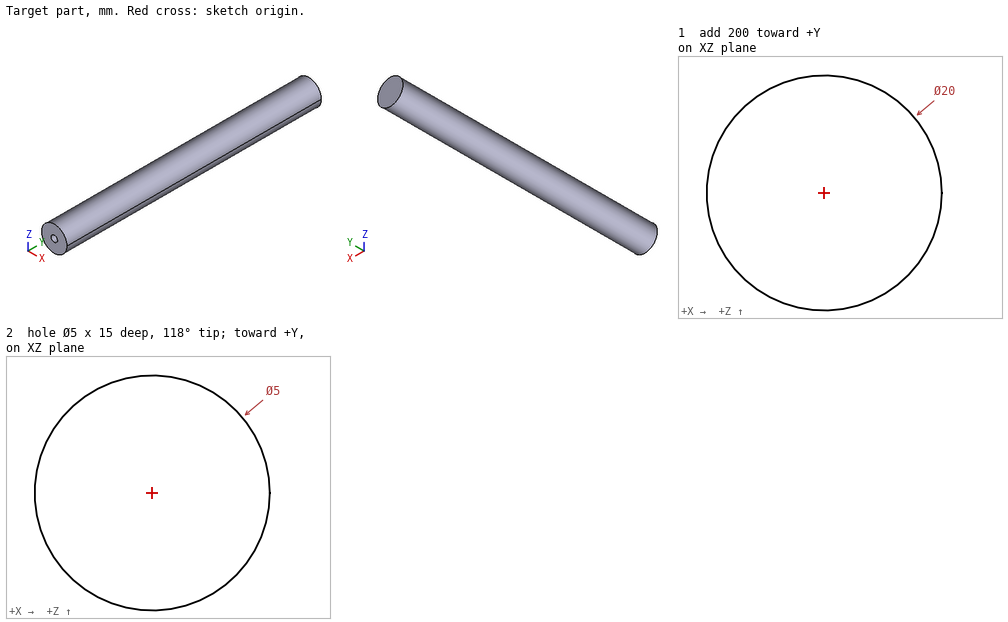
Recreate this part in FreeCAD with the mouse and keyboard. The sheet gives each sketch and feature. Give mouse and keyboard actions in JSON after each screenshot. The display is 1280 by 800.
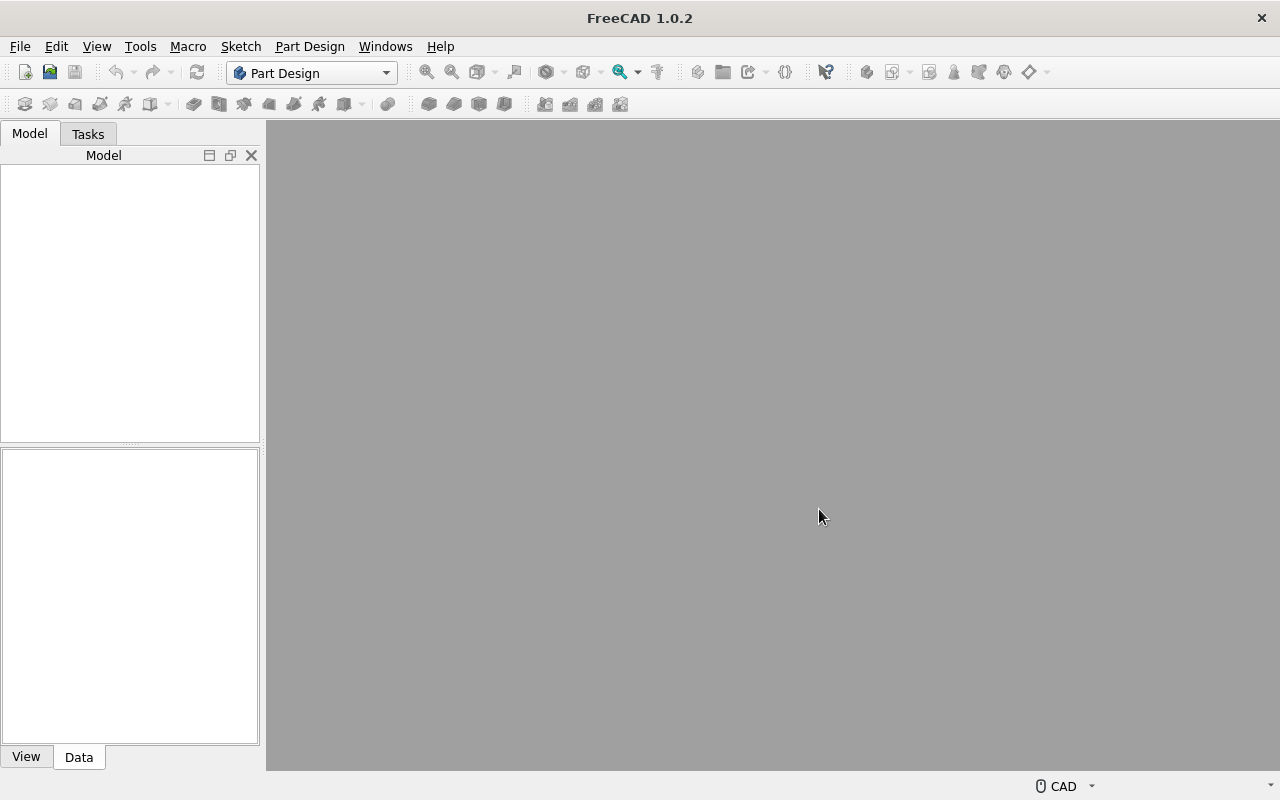
{"action": "key", "text": "ctrl+n"}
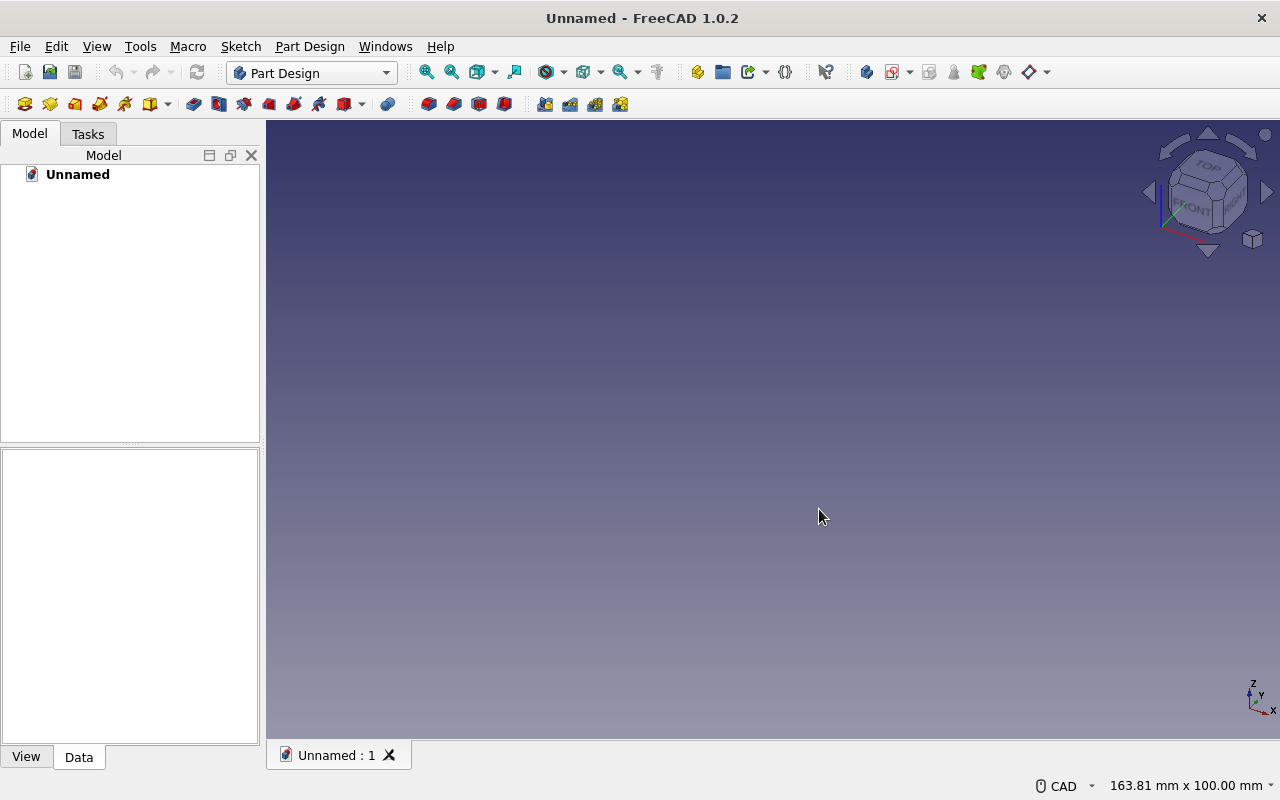
{"action": "left_click", "coordinate": [892, 72]}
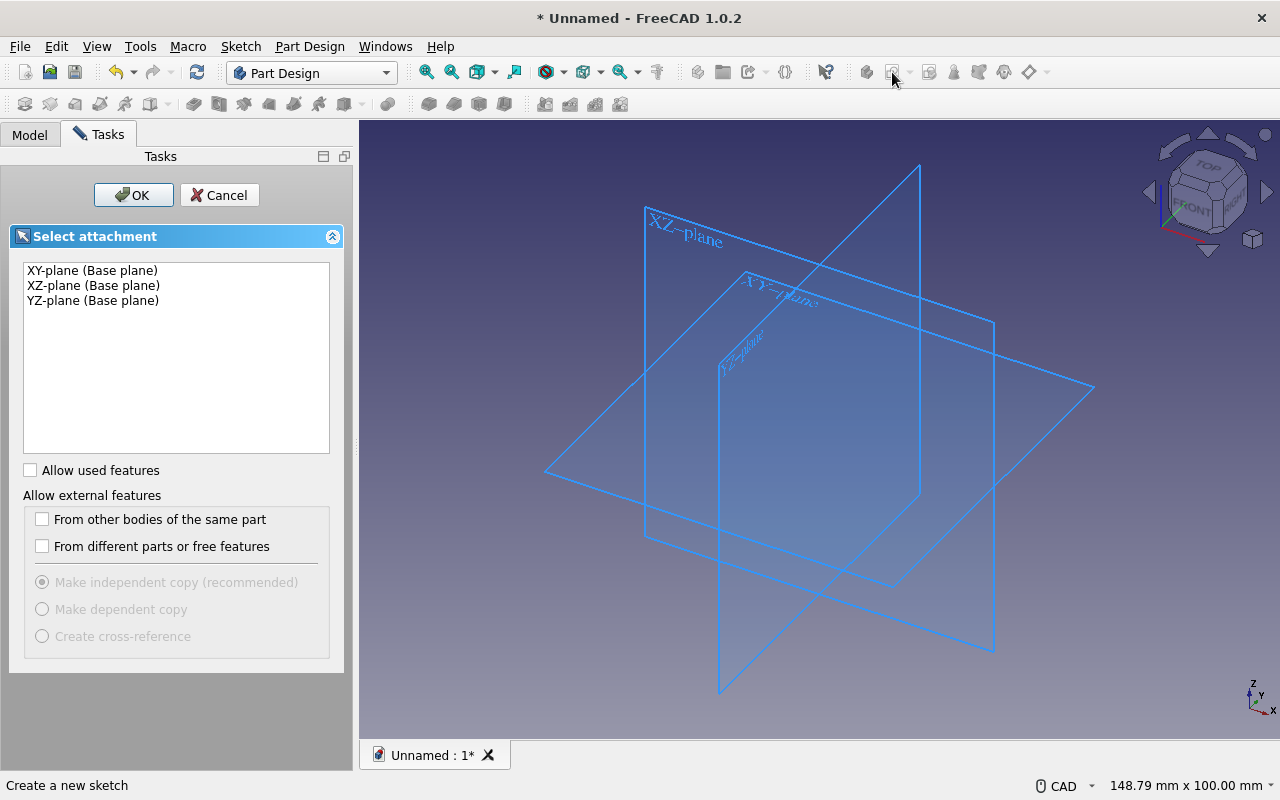
{"action": "left_click", "coordinate": [84, 286]}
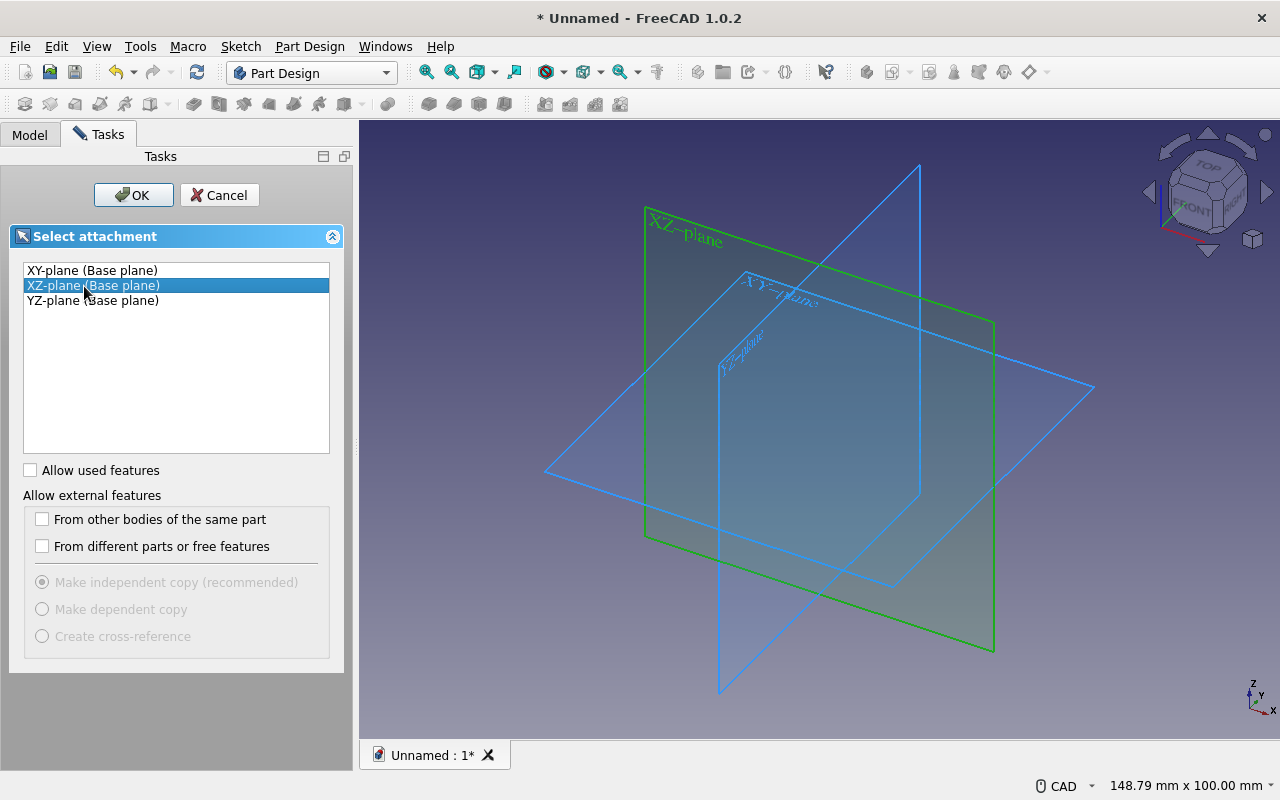
{"action": "left_click", "coordinate": [134, 195]}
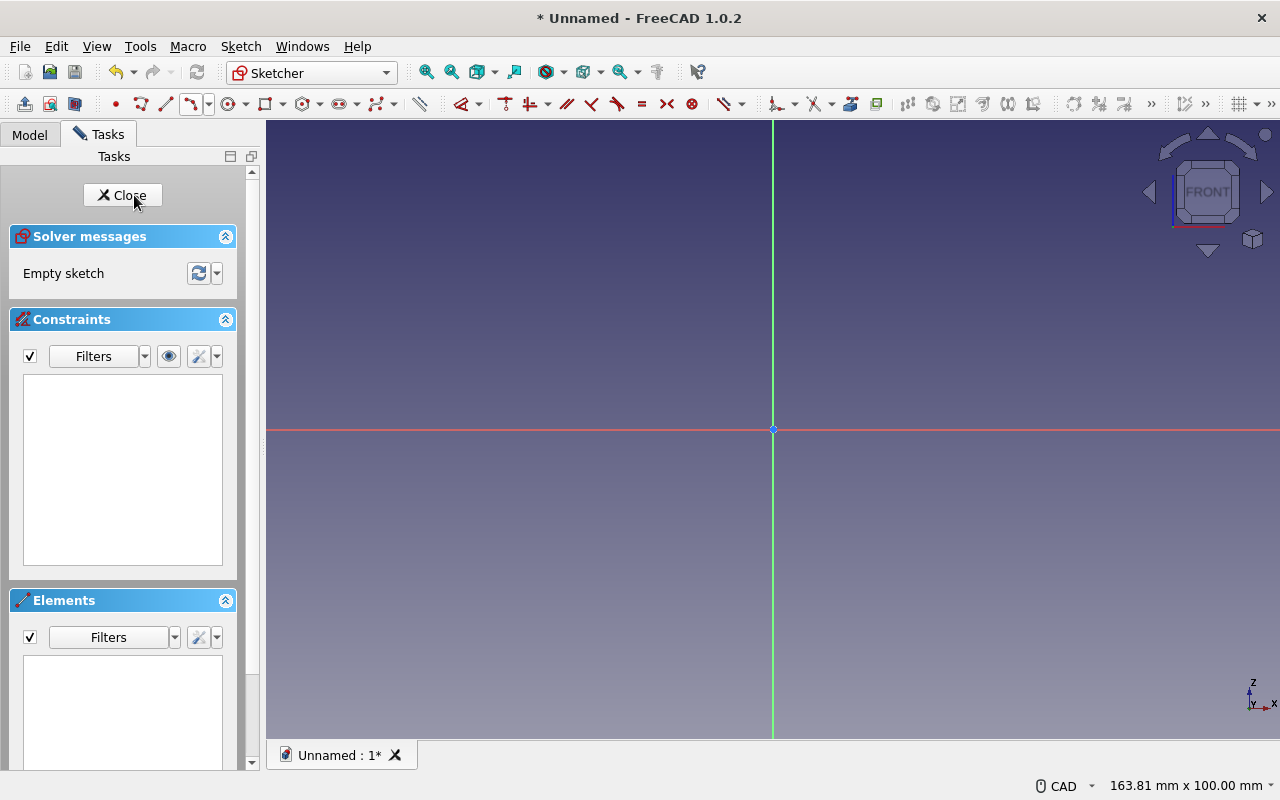
{"action": "scroll", "coordinate": [803, 430], "scroll_direction": "up", "scroll_amount": 6}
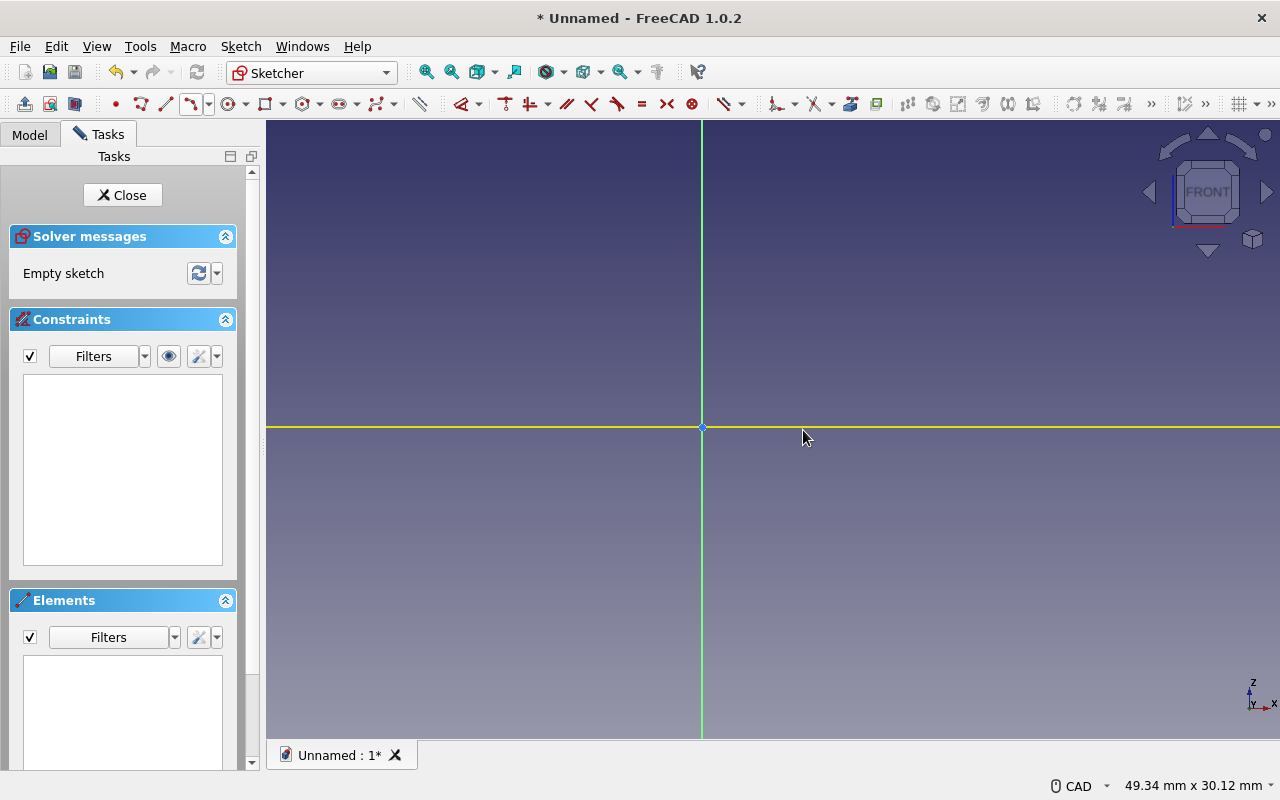
{"action": "left_click", "coordinate": [228, 104]}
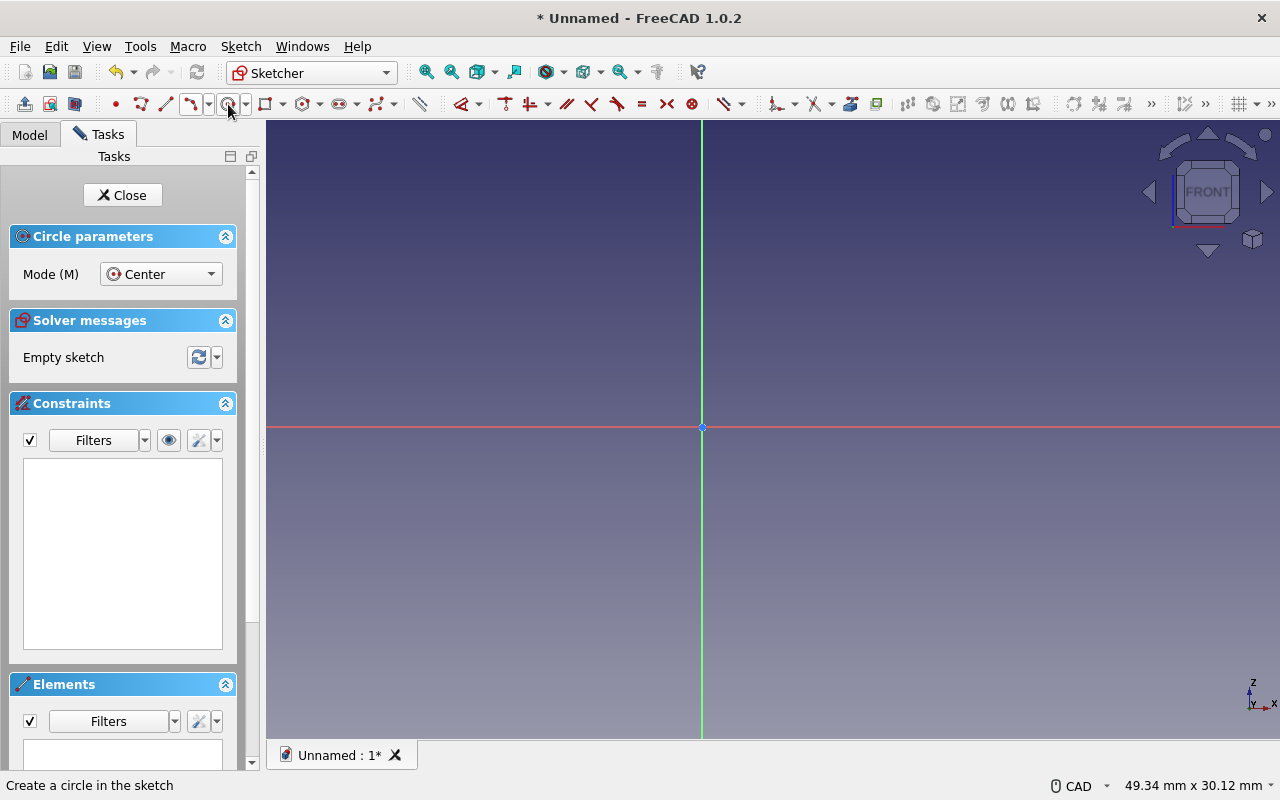
{"action": "left_click", "coordinate": [702, 427]}
{"action": "mouse_move", "coordinate": [847, 282]}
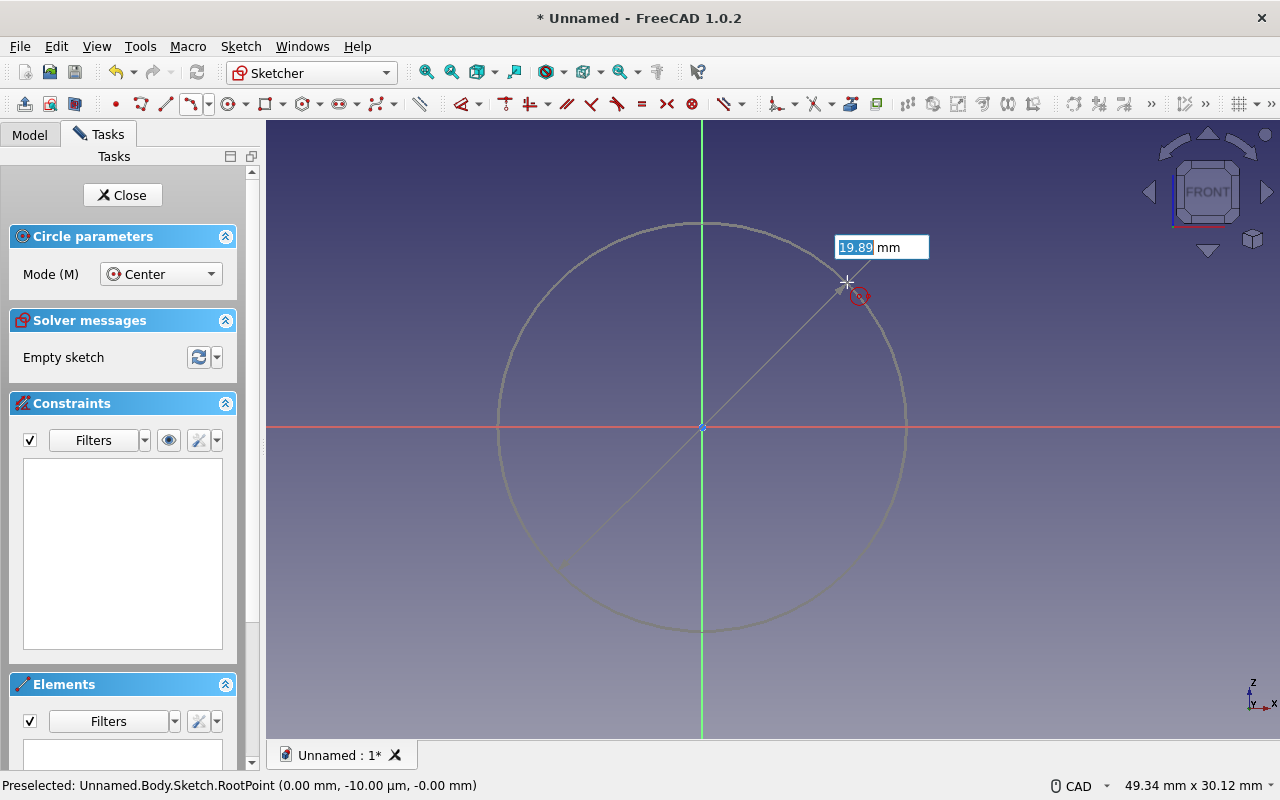
{"action": "type", "text": "20"}
{"action": "key", "text": "Return"}
{"action": "key", "text": "Escape"}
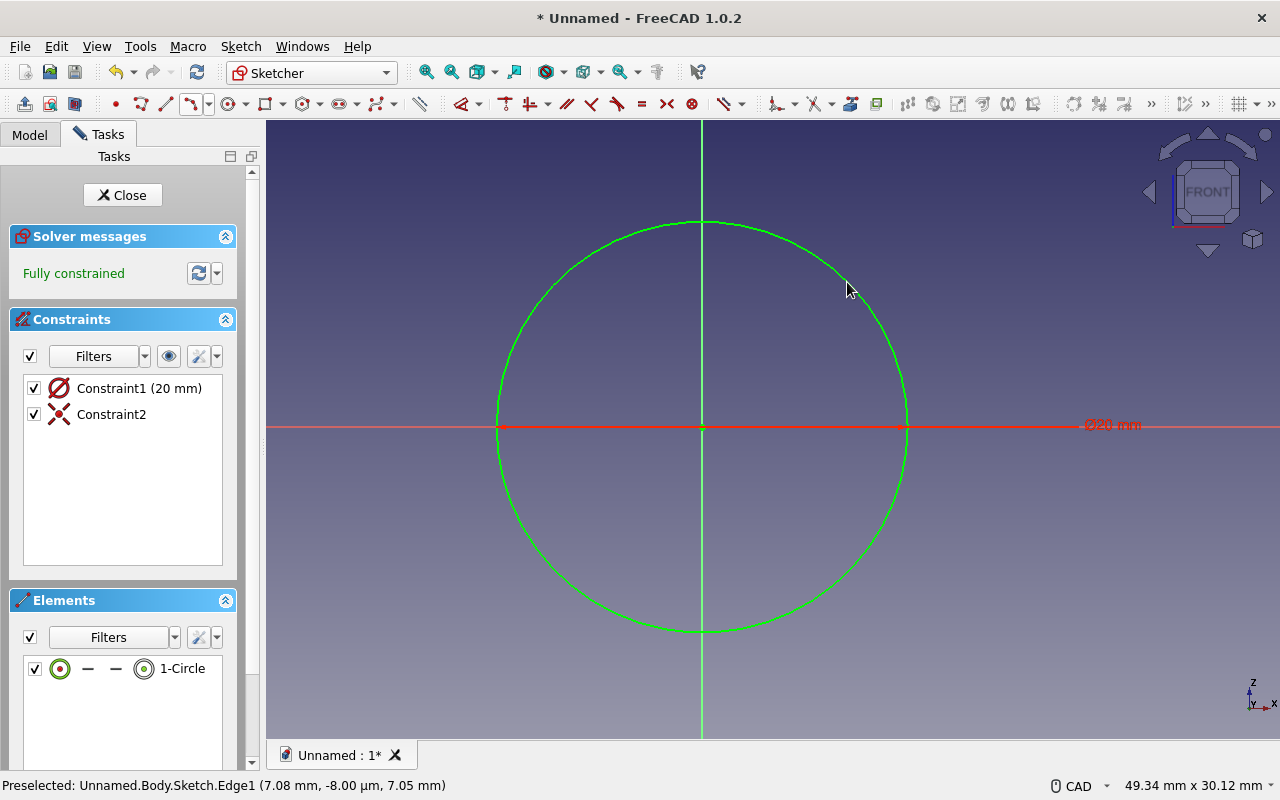
{"action": "left_click", "coordinate": [123, 195]}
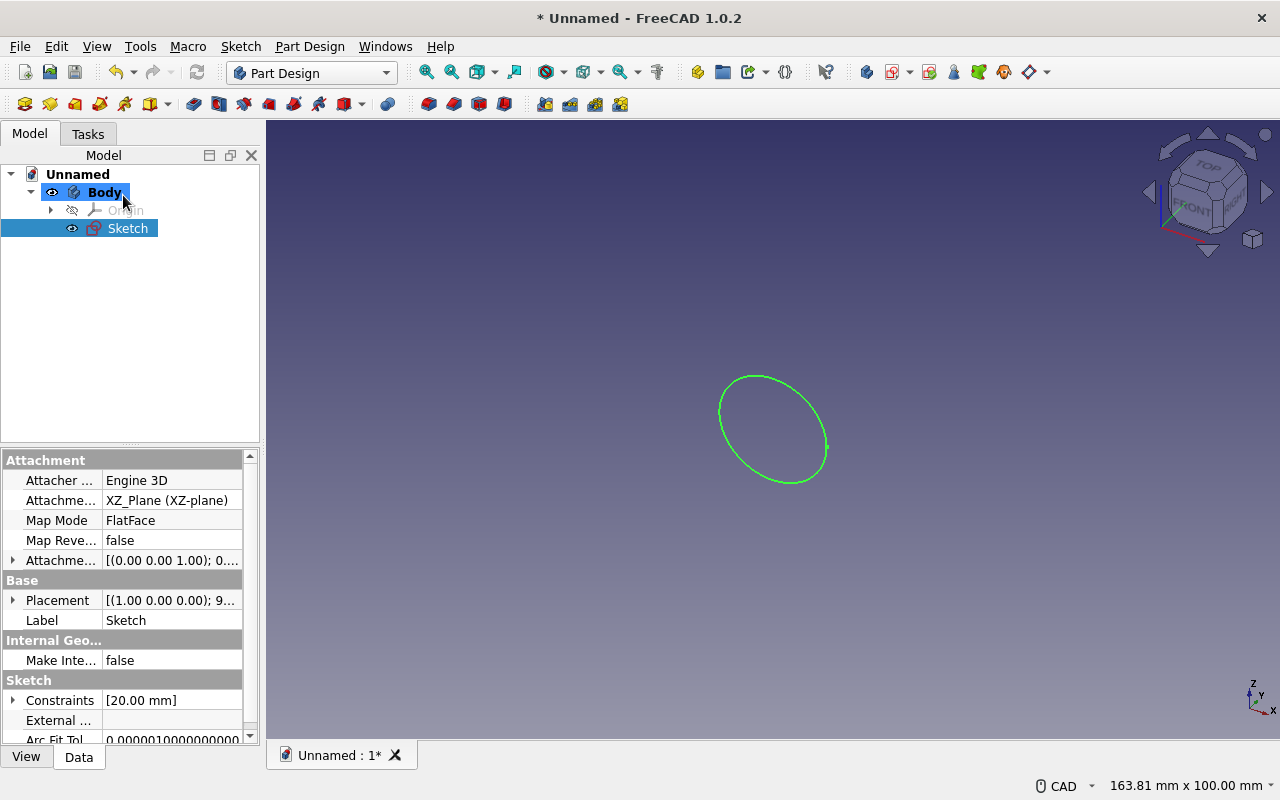
{"action": "left_click", "coordinate": [25, 104]}